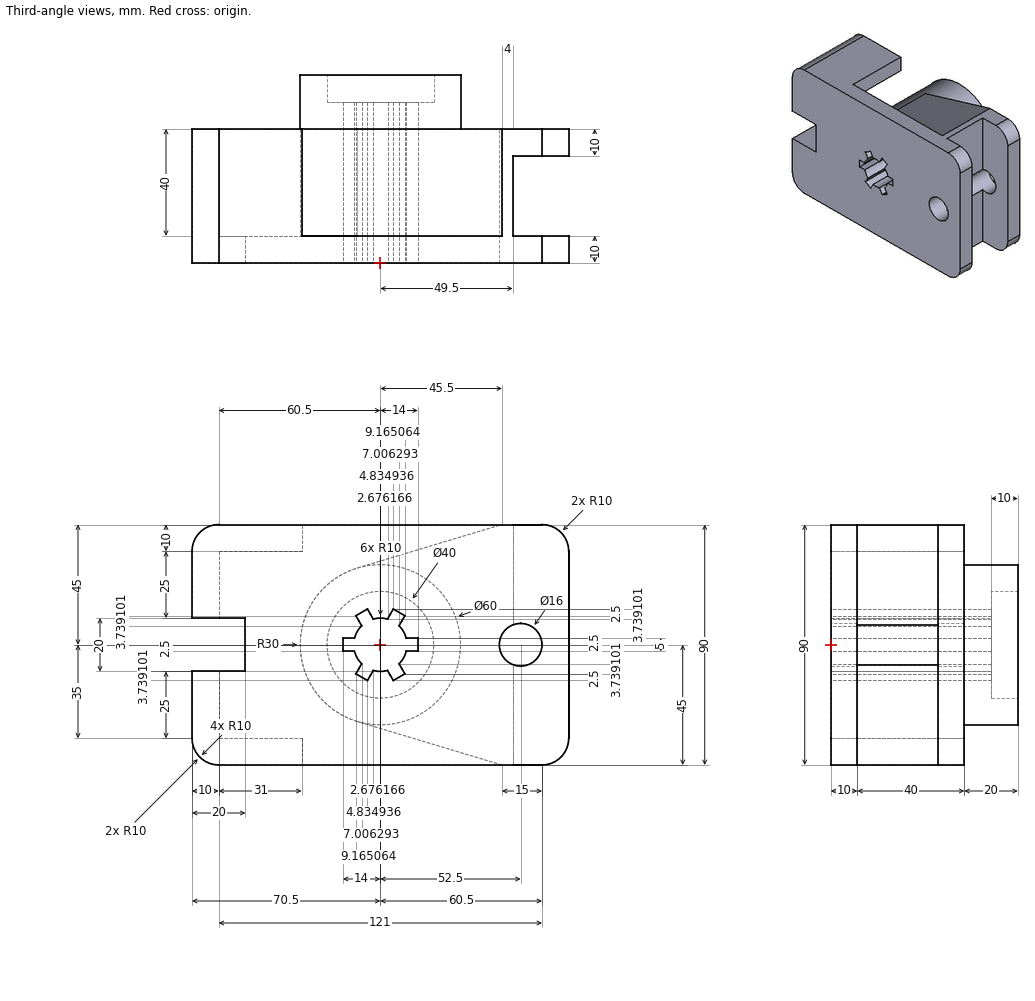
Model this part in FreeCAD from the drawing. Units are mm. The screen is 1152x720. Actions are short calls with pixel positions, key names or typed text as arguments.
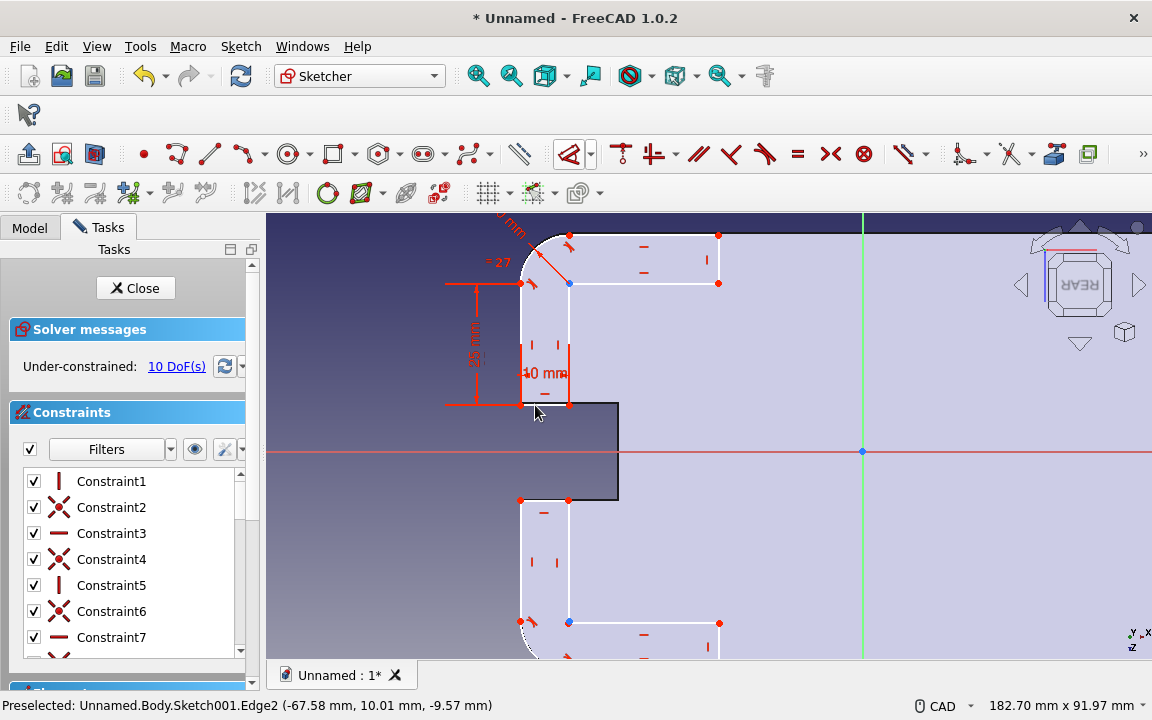
click(569, 369)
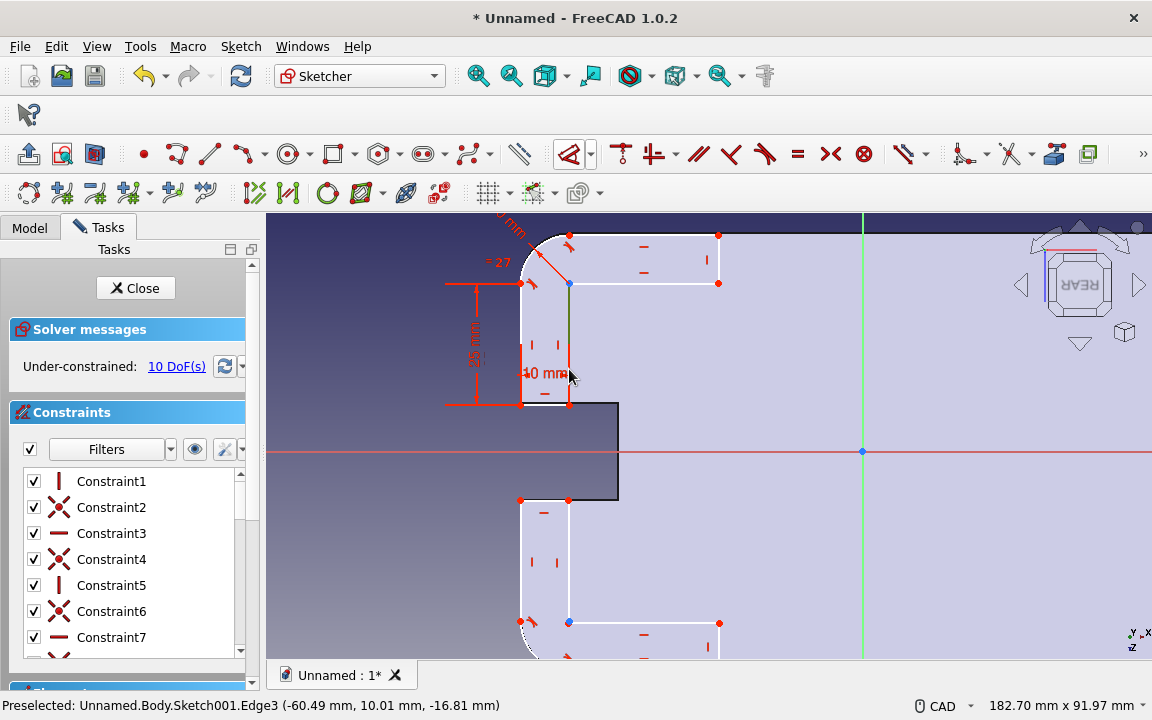
click(590, 154)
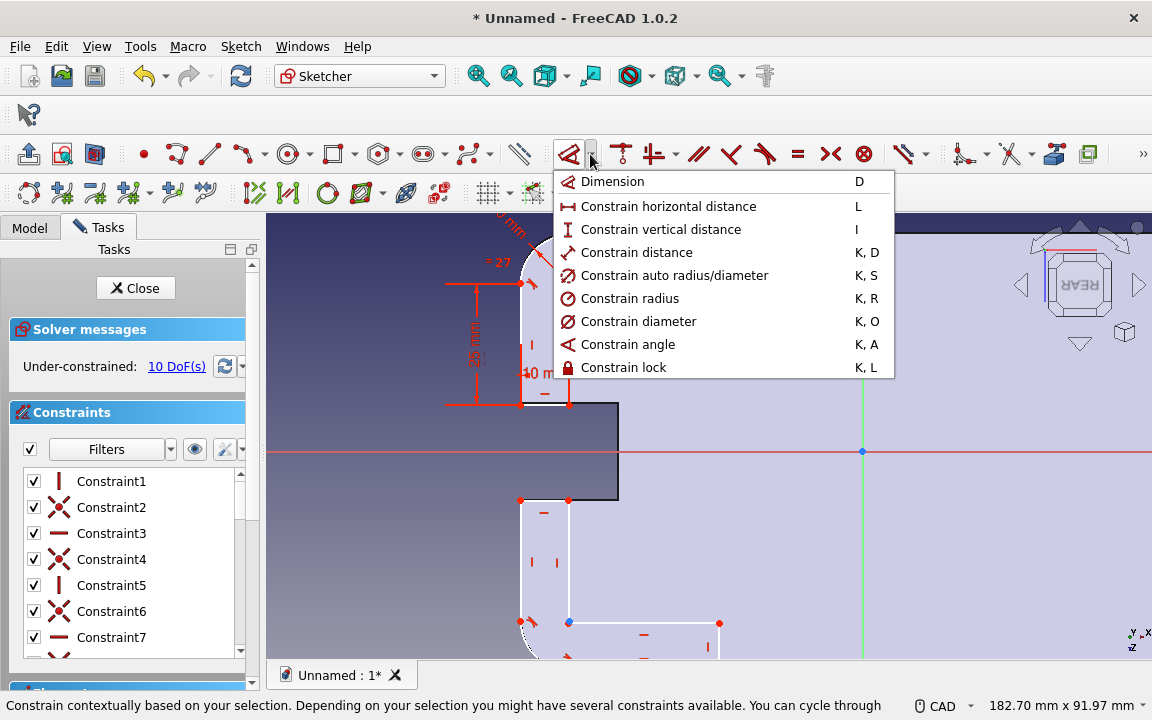
click(724, 230)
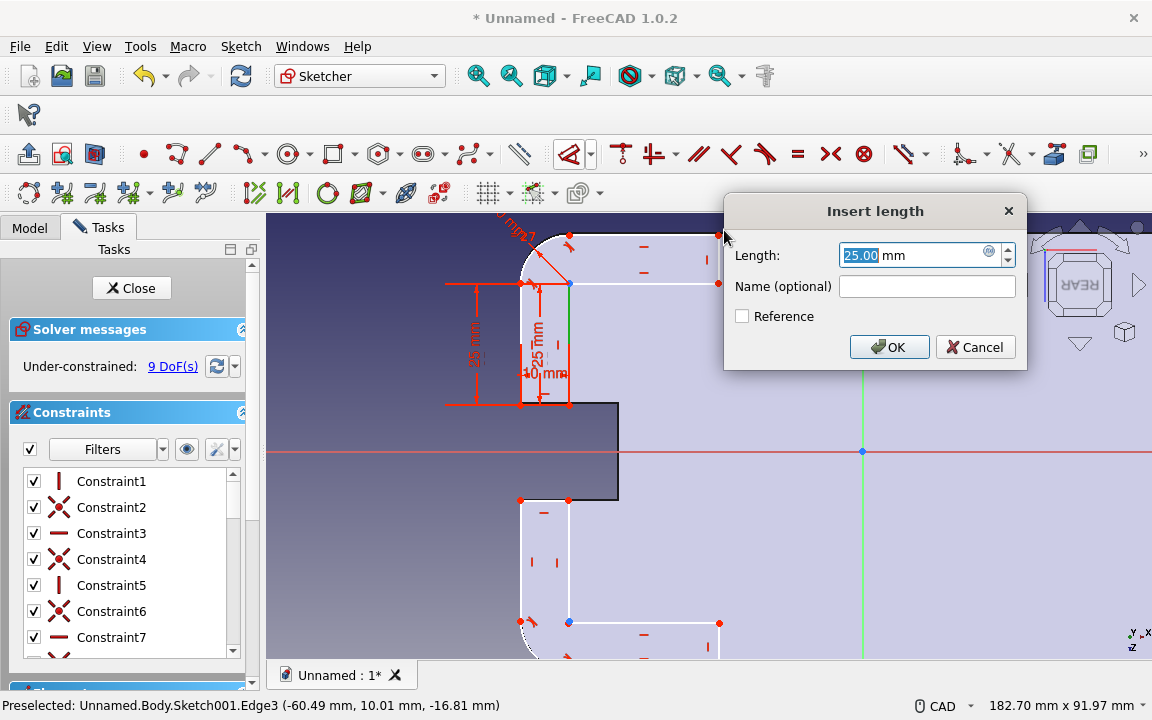
text(25)
key(Return)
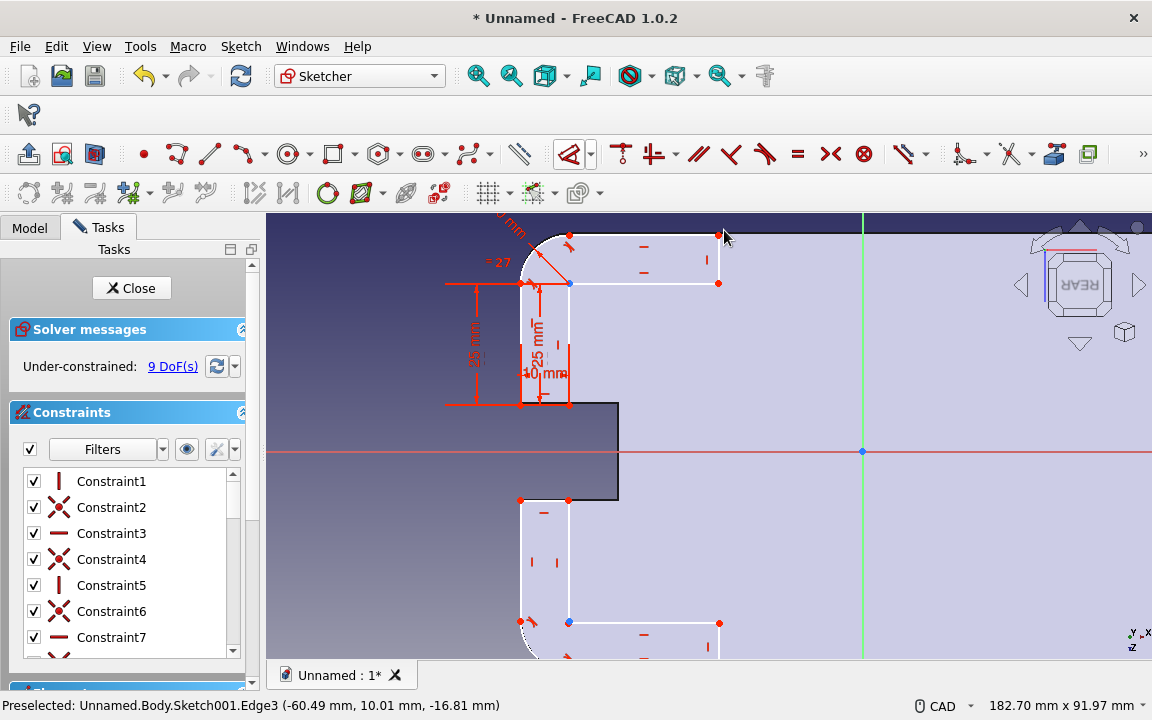
click(614, 284)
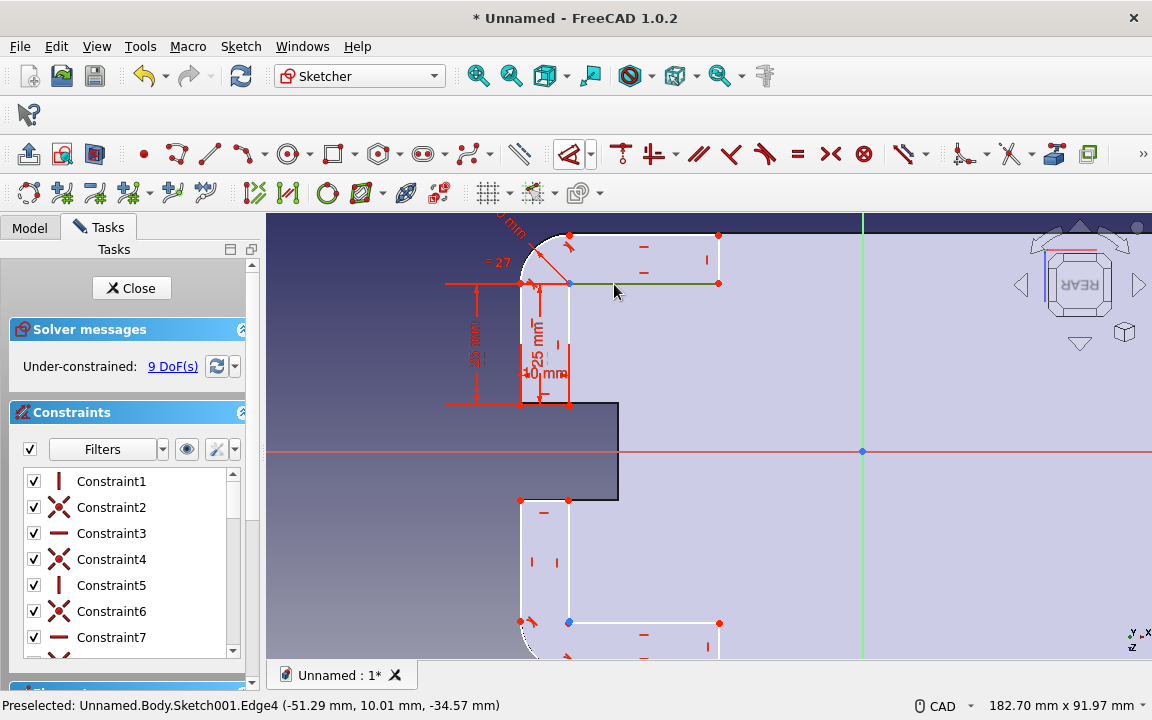
key(l)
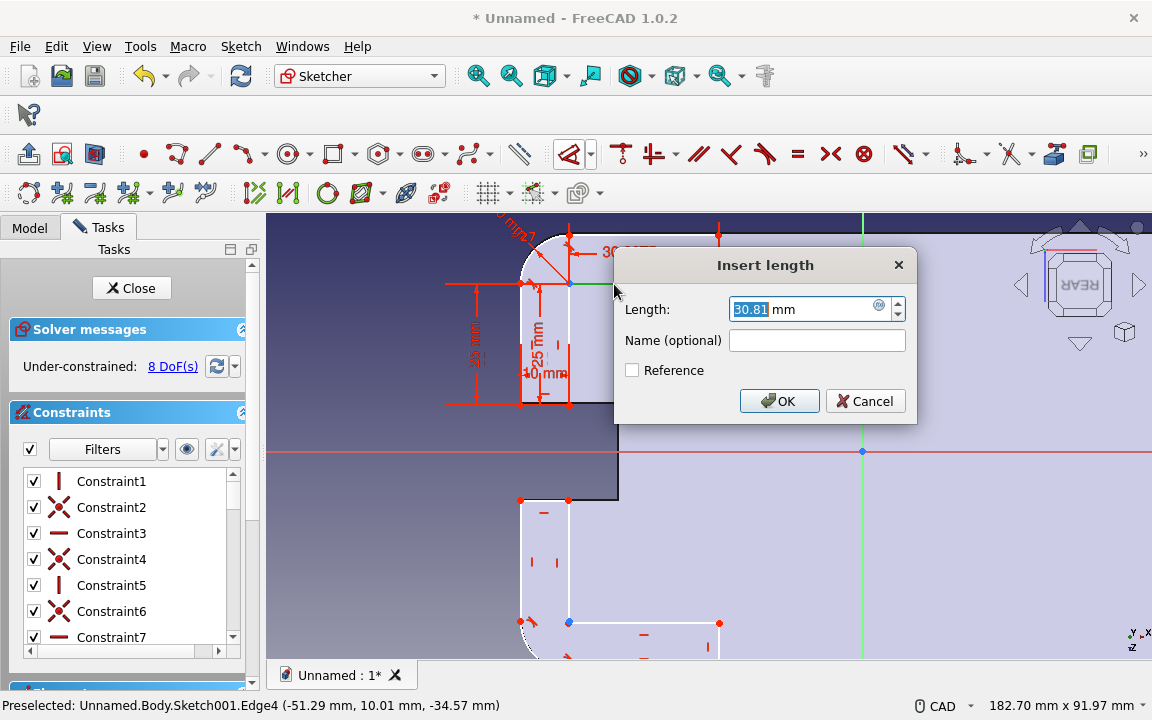
text(31)
key(Return)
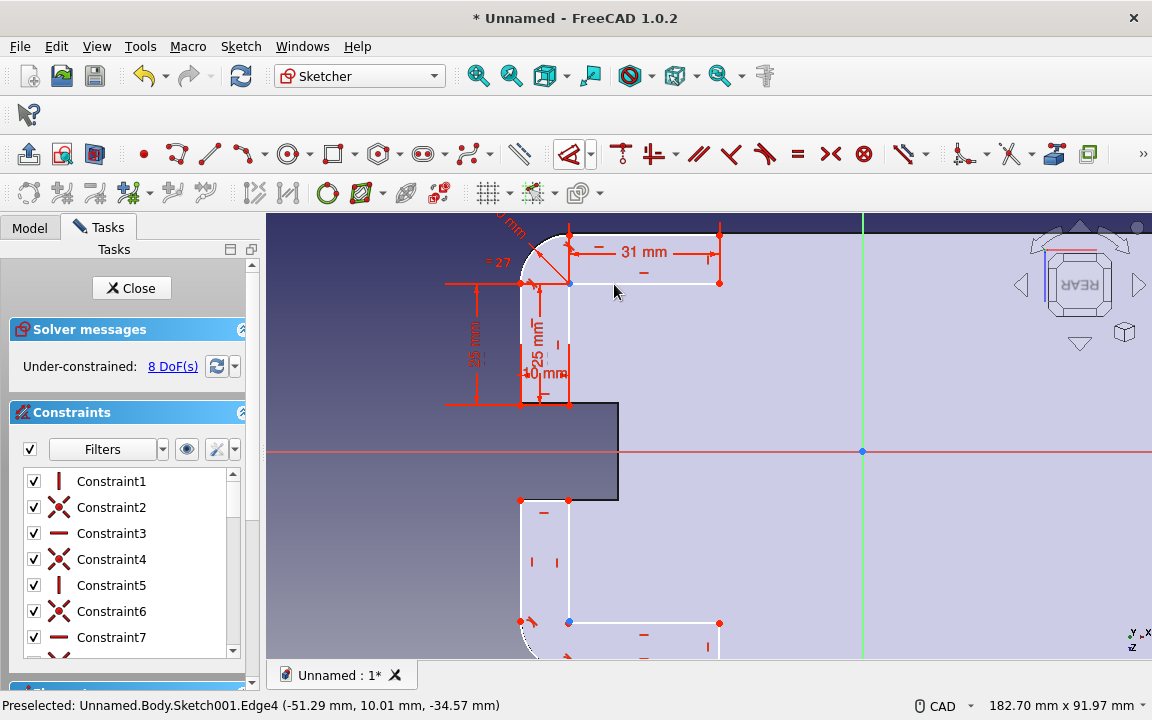
scroll(536, 404, down, 2)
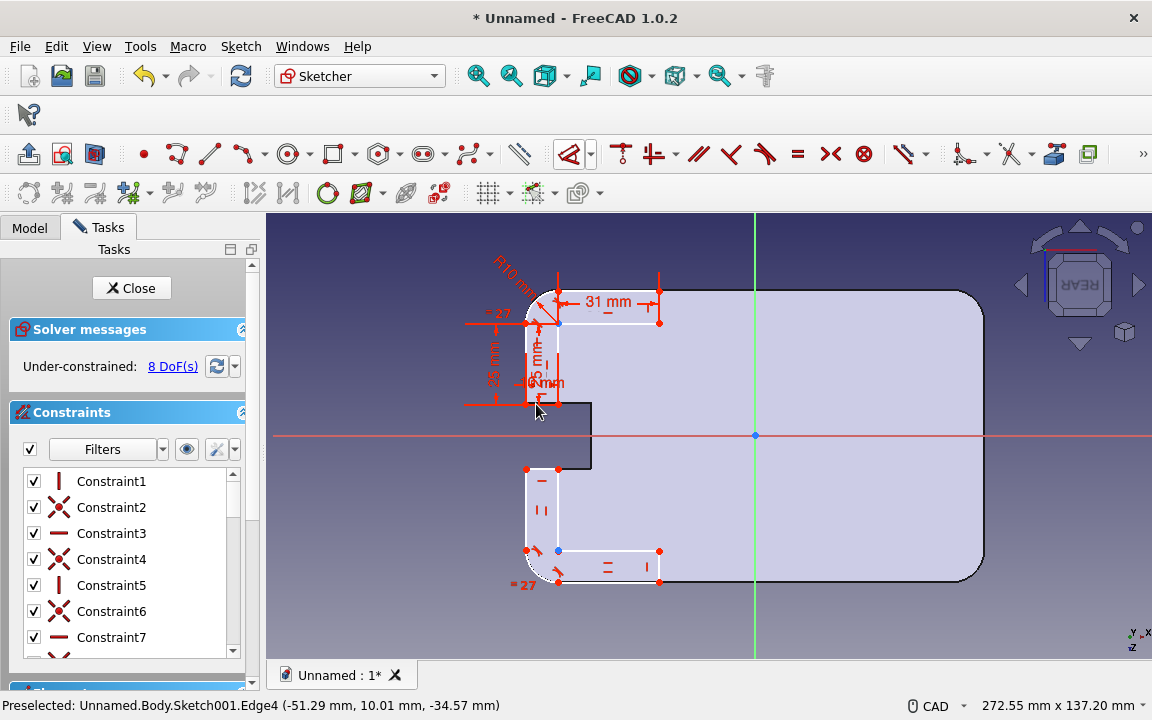
click(589, 583)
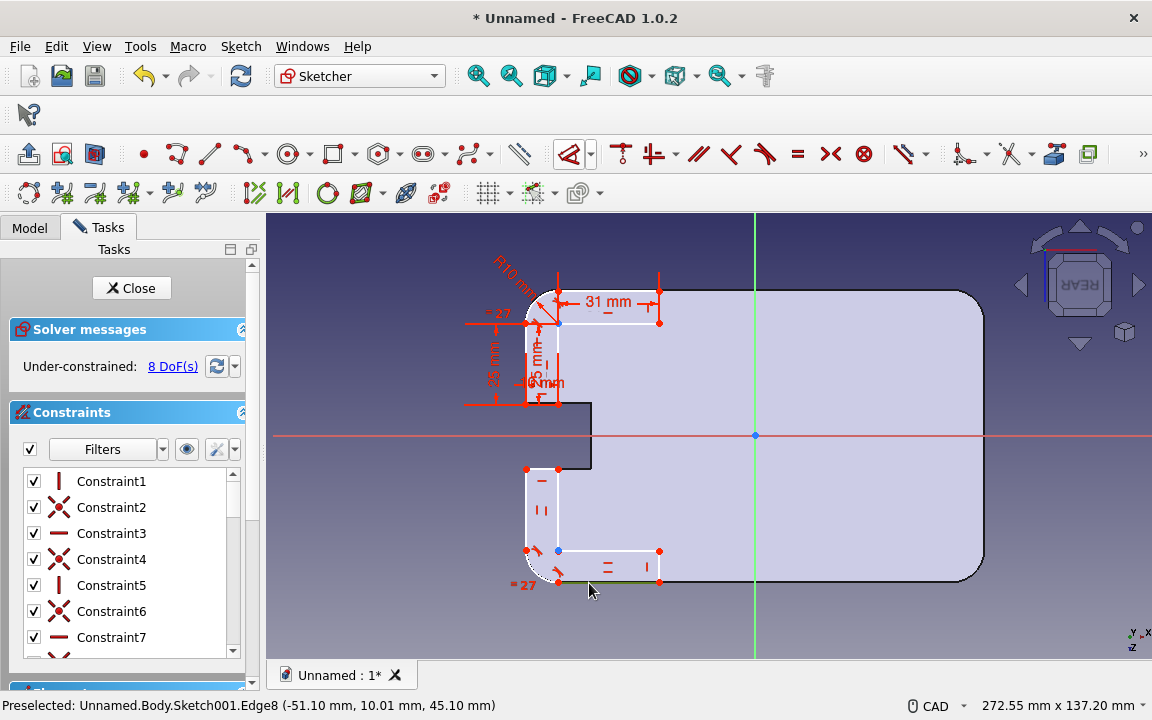
key(l)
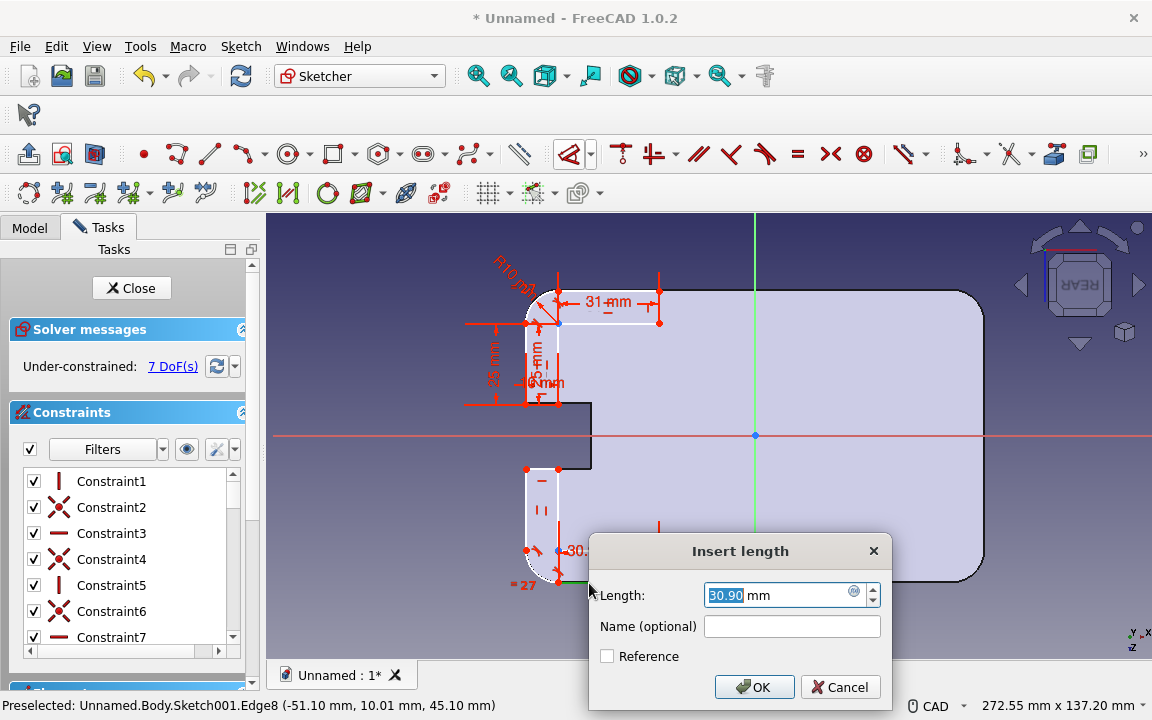
text(31)
key(Return)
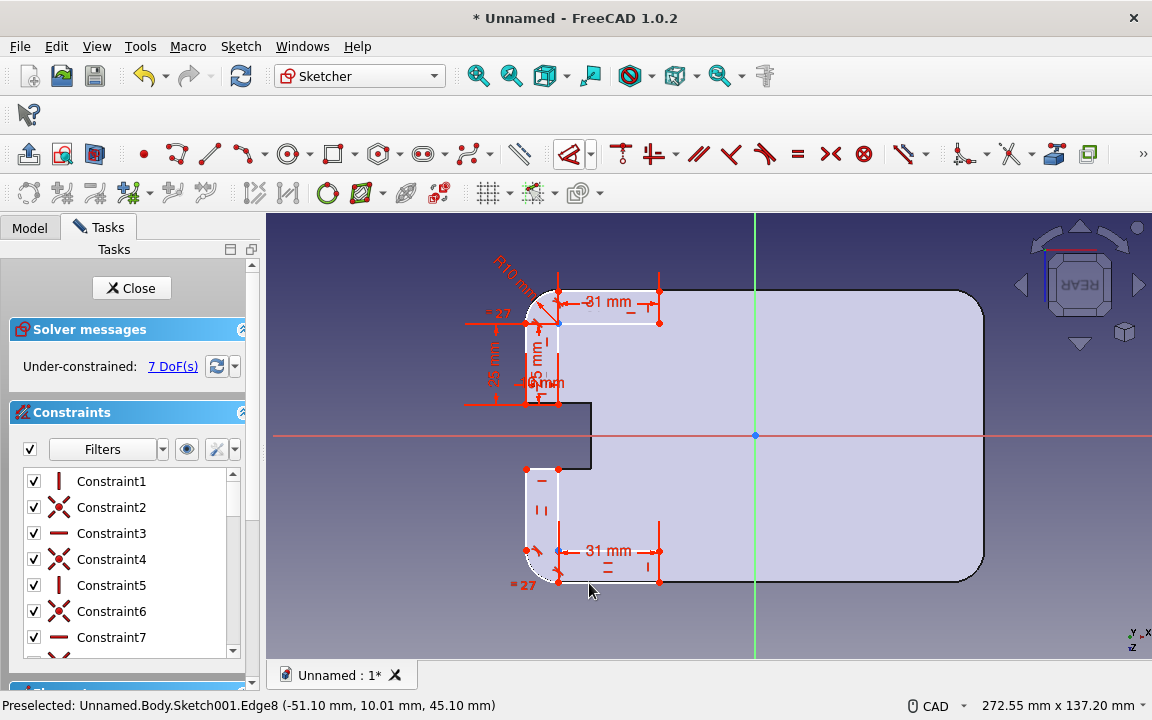
scroll(659, 573, up, 2)